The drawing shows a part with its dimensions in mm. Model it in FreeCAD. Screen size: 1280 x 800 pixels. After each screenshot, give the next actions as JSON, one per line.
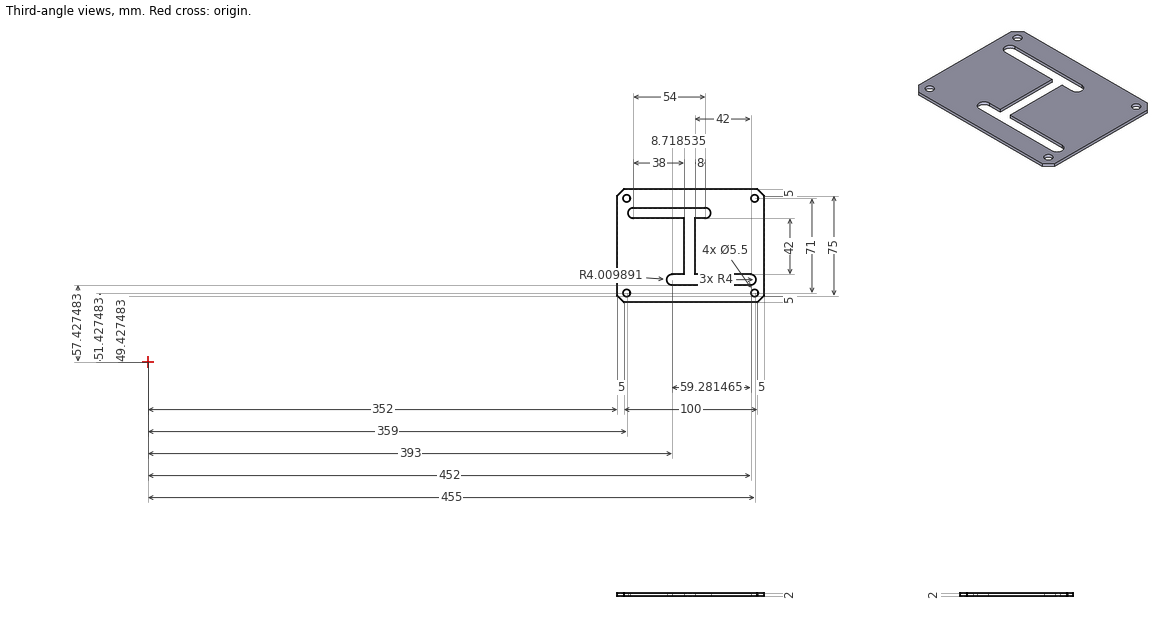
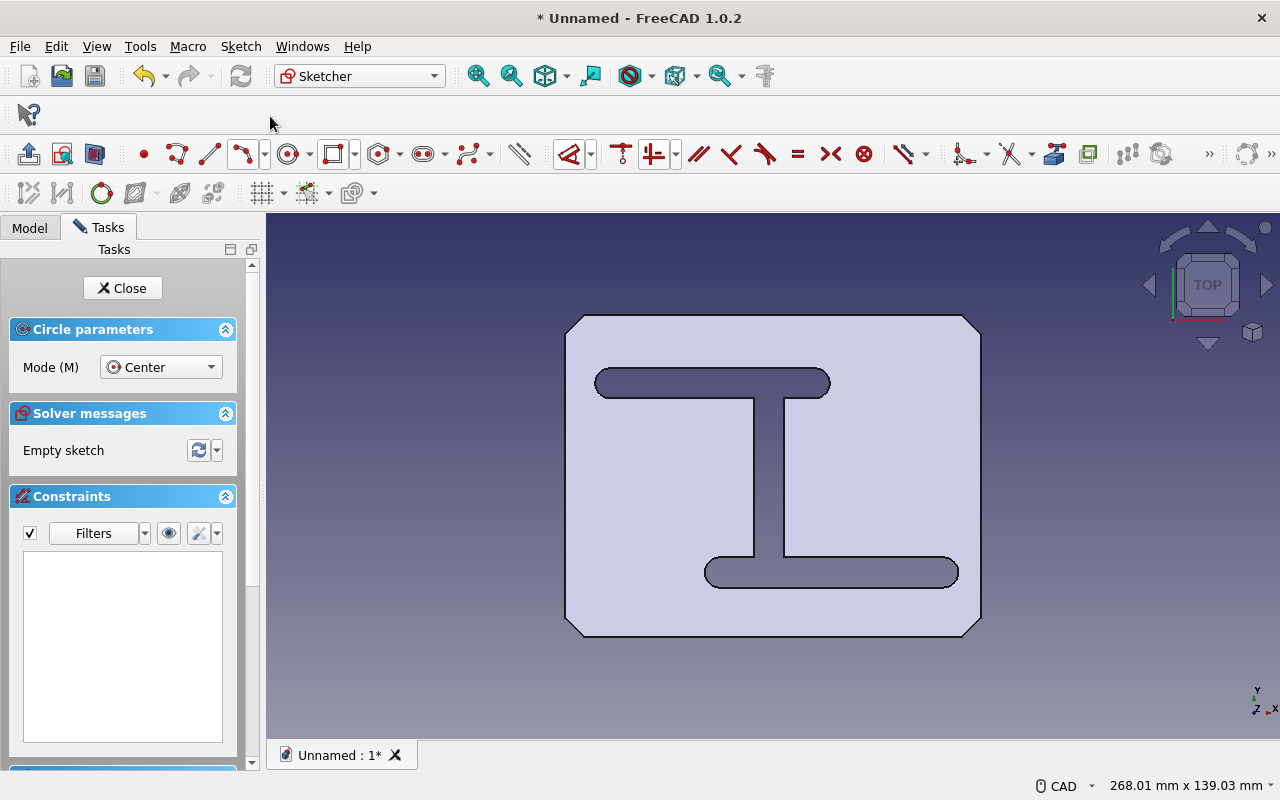
{"action": "scroll", "coordinate": [955, 610], "scroll_direction": "up", "scroll_amount": 4}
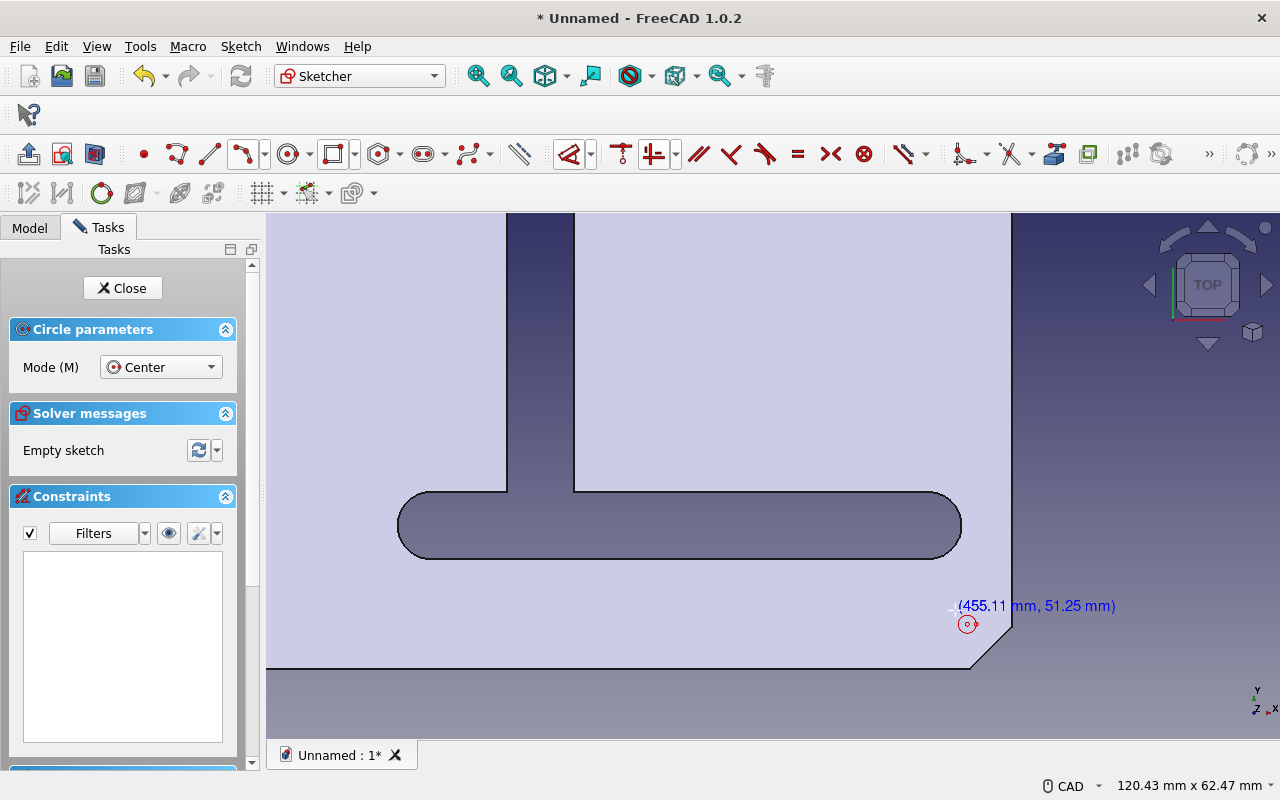
{"action": "left_click", "coordinate": [953, 610]}
{"action": "left_click", "coordinate": [970, 593]}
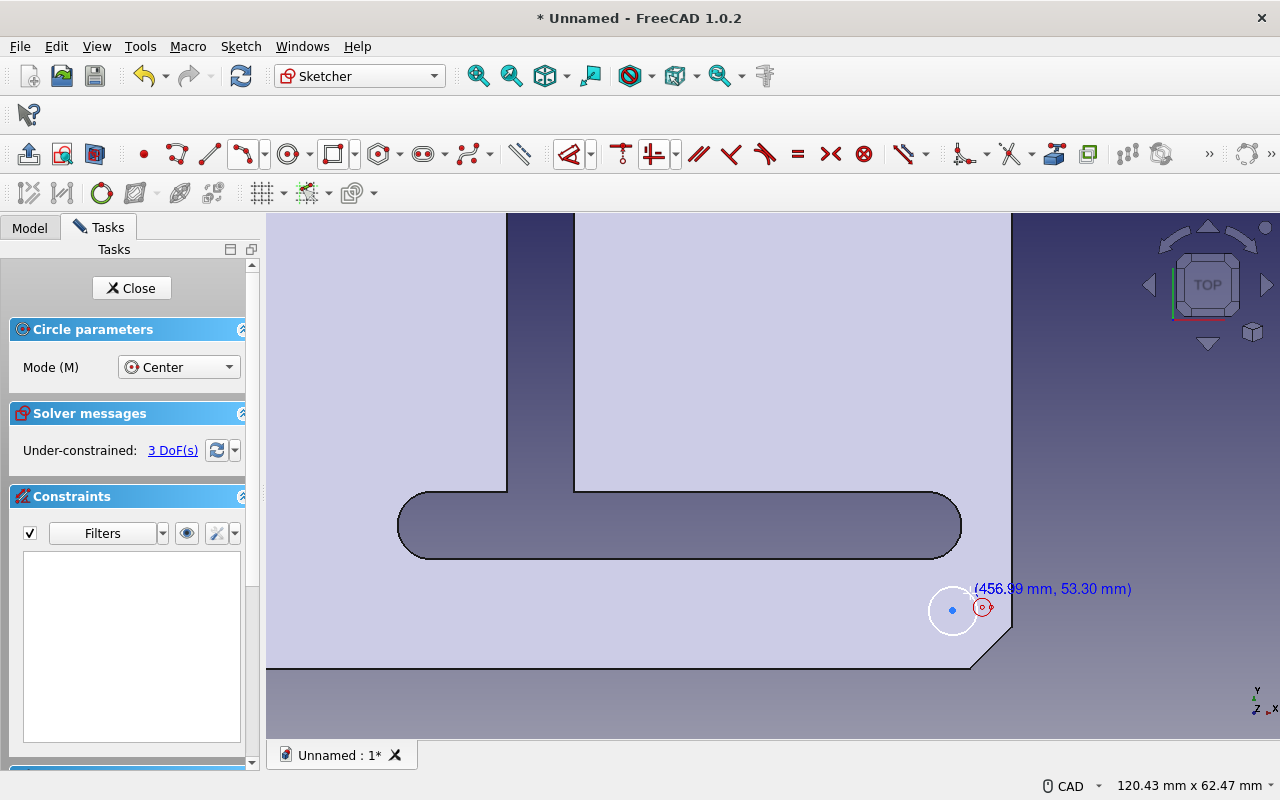
{"action": "scroll", "coordinate": [894, 677], "scroll_direction": "down", "scroll_amount": 3}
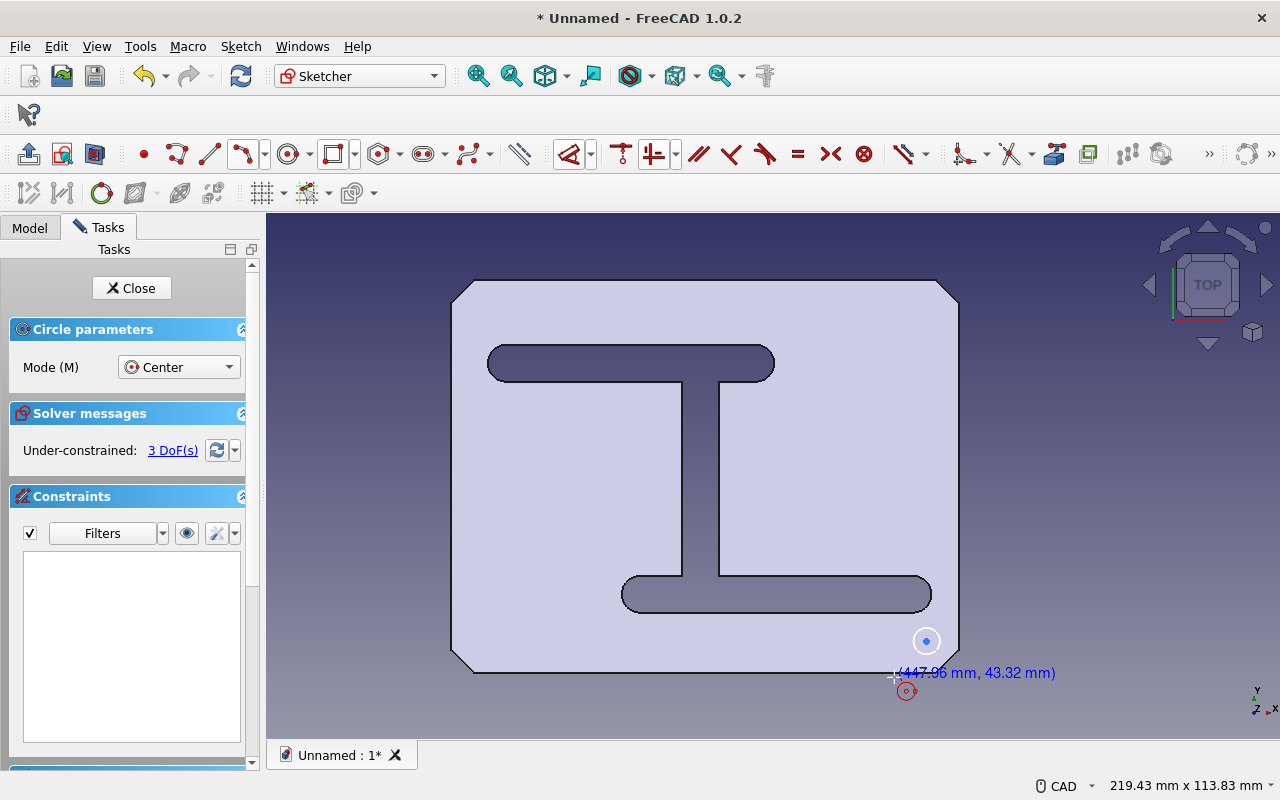
{"action": "scroll", "coordinate": [483, 640], "scroll_direction": "up", "scroll_amount": 3}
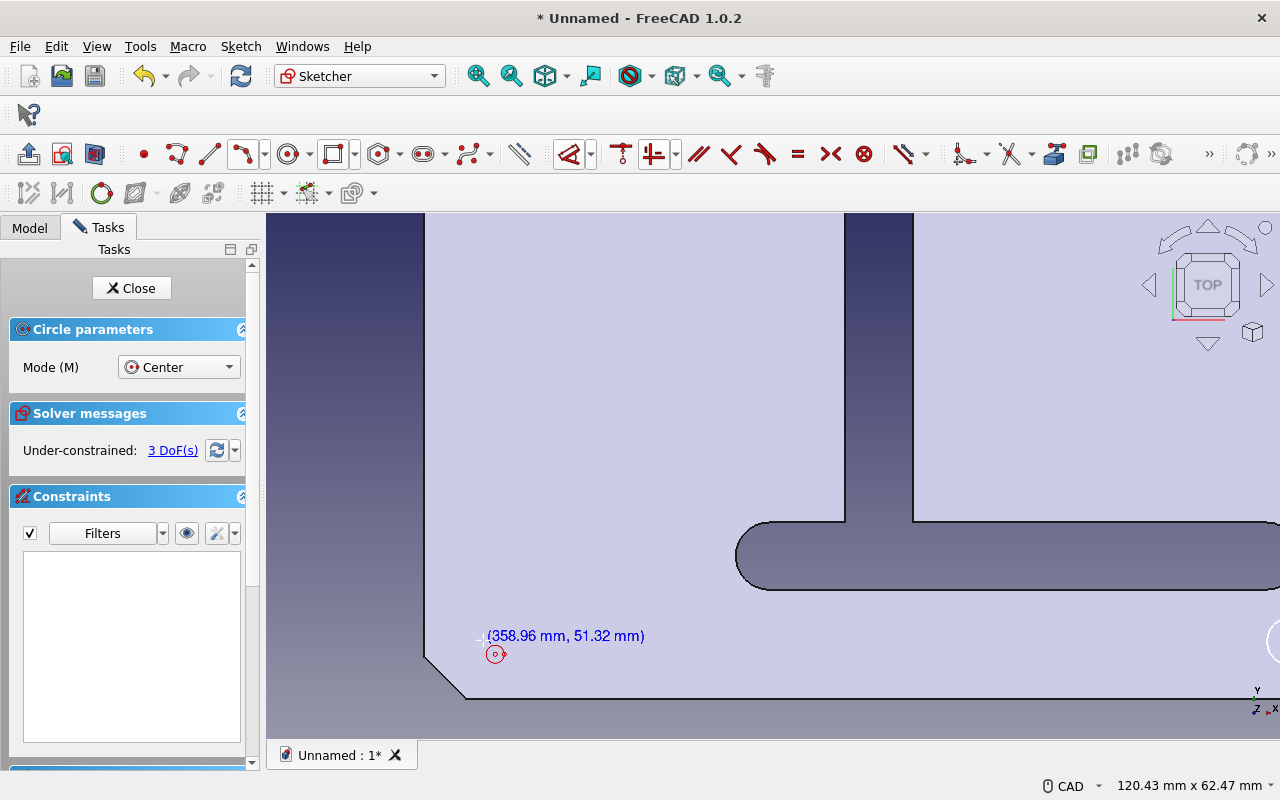
{"action": "left_click", "coordinate": [483, 640]}
{"action": "left_click", "coordinate": [500, 624]}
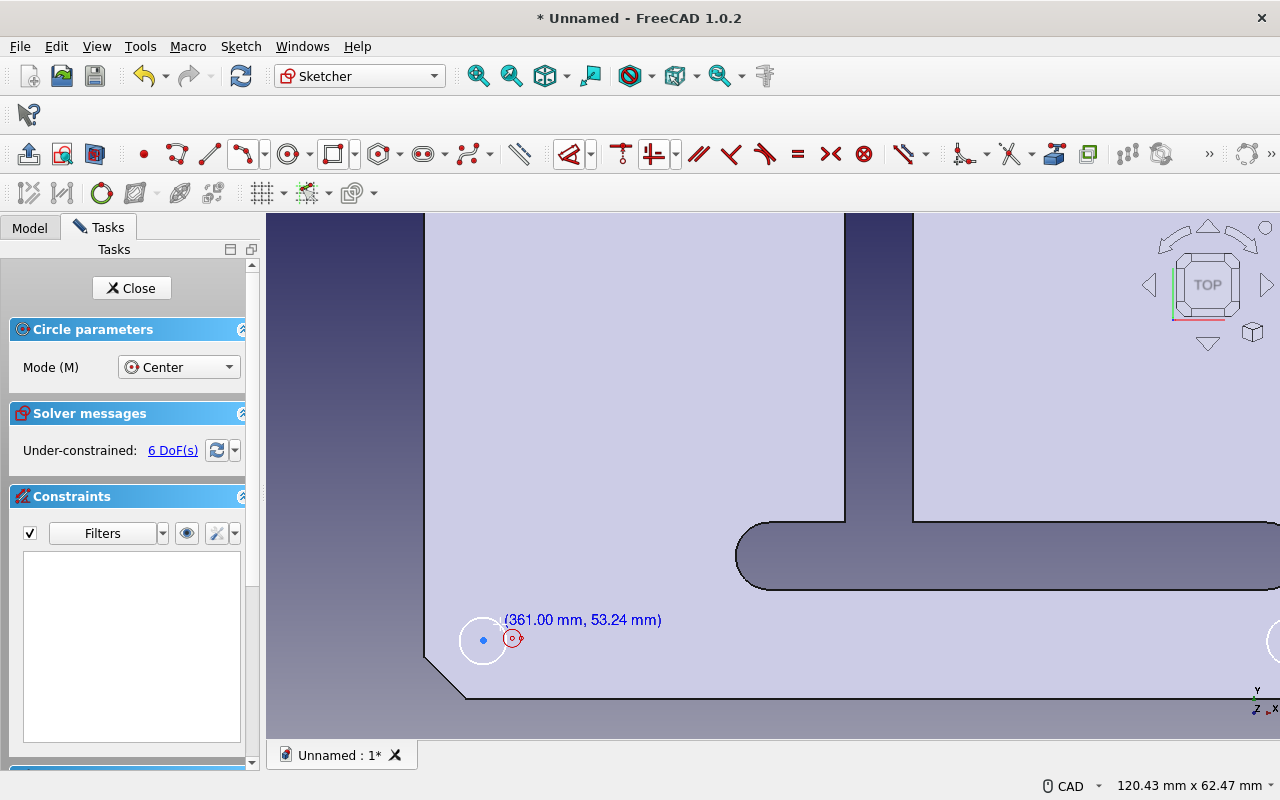
{"action": "scroll", "coordinate": [482, 640], "scroll_direction": "down", "scroll_amount": 3}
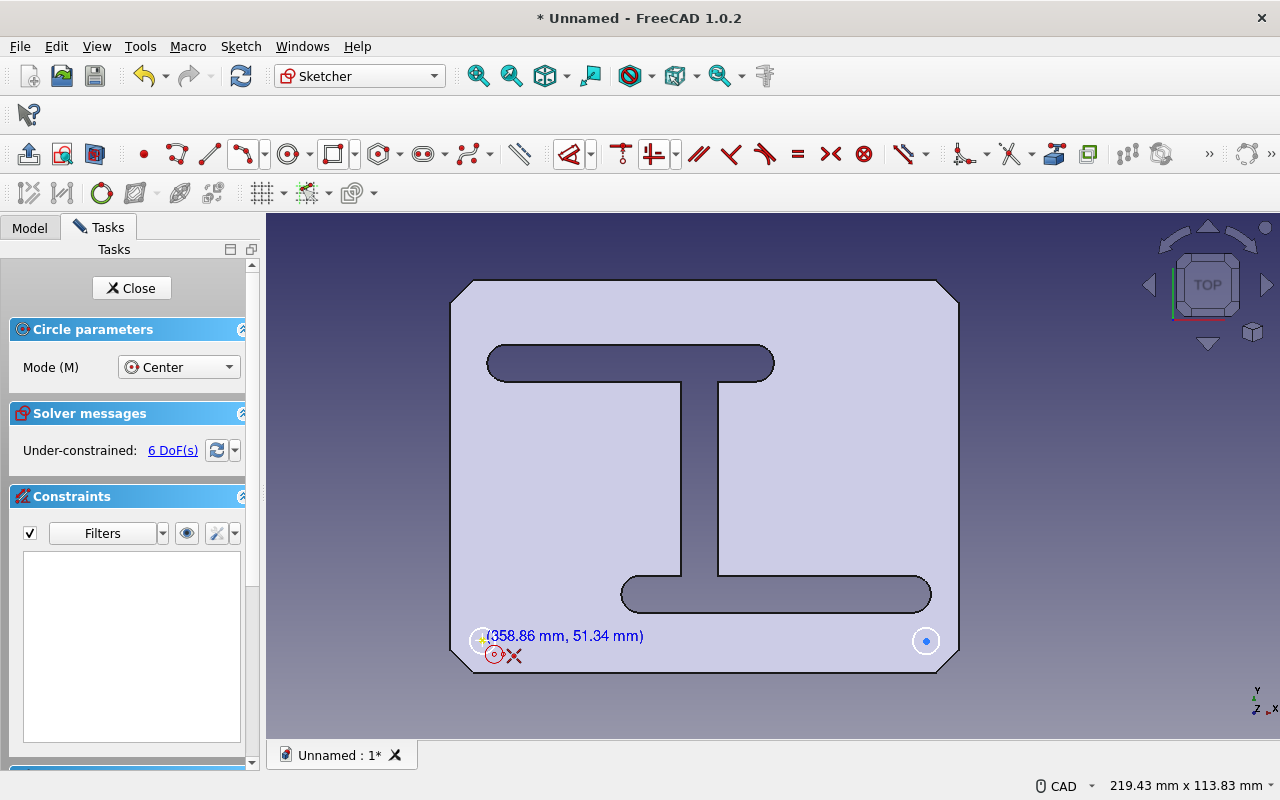
{"action": "scroll", "coordinate": [926, 312], "scroll_direction": "up", "scroll_amount": 3}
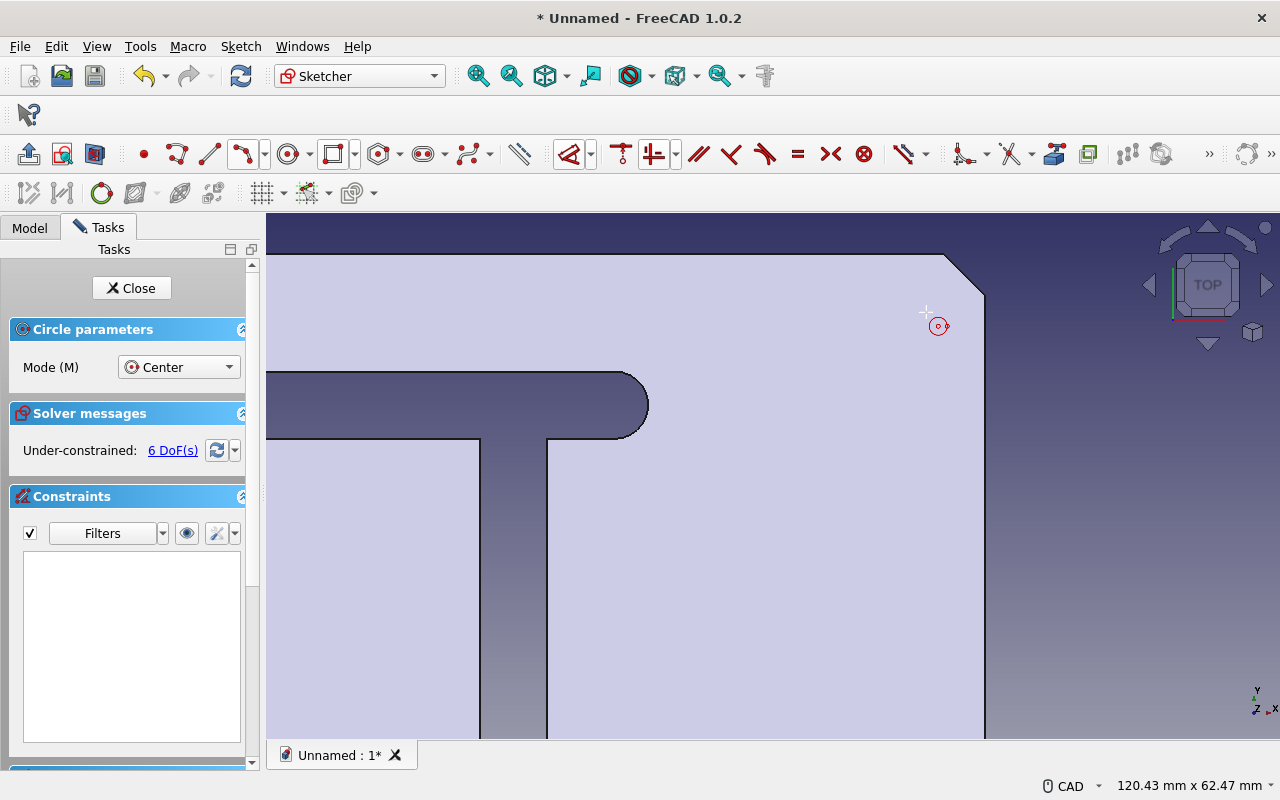
{"action": "left_click", "coordinate": [926, 313]}
{"action": "left_click", "coordinate": [942, 296]}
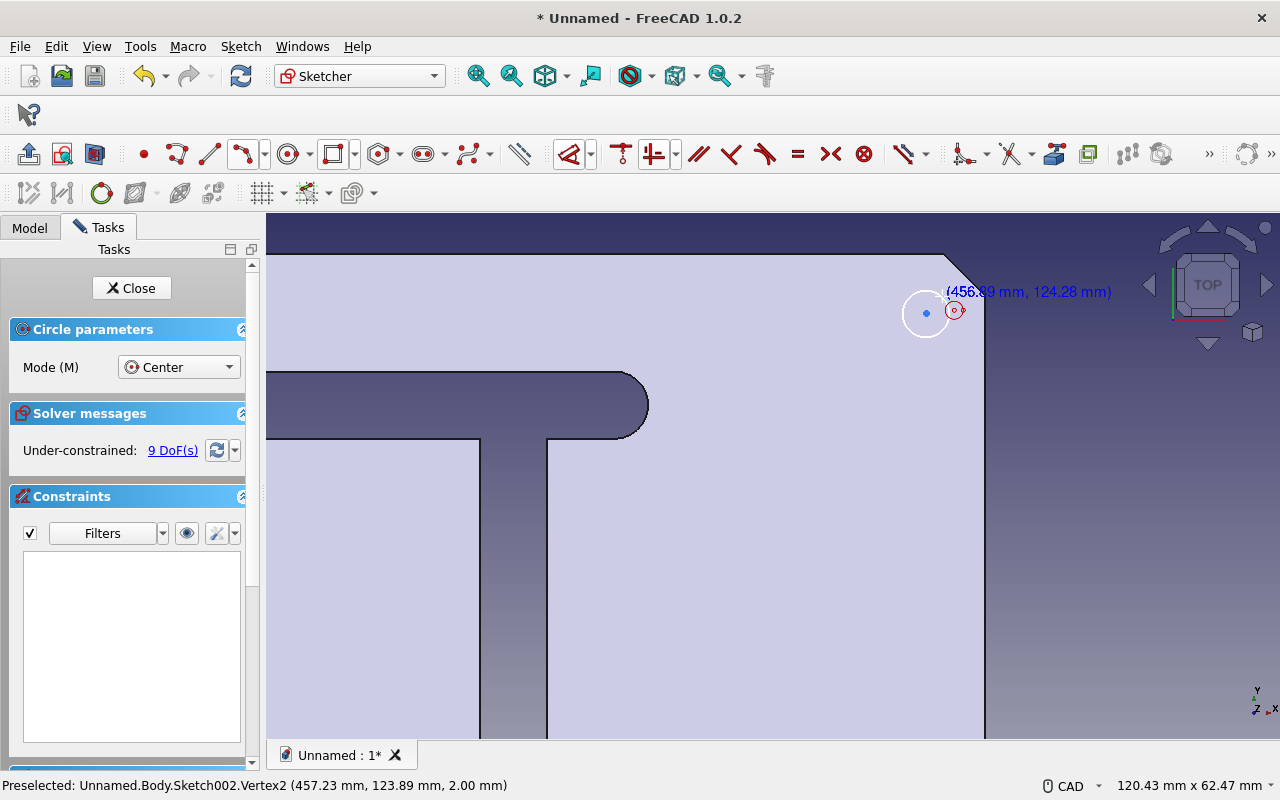
{"action": "scroll", "coordinate": [927, 311], "scroll_direction": "down", "scroll_amount": 3}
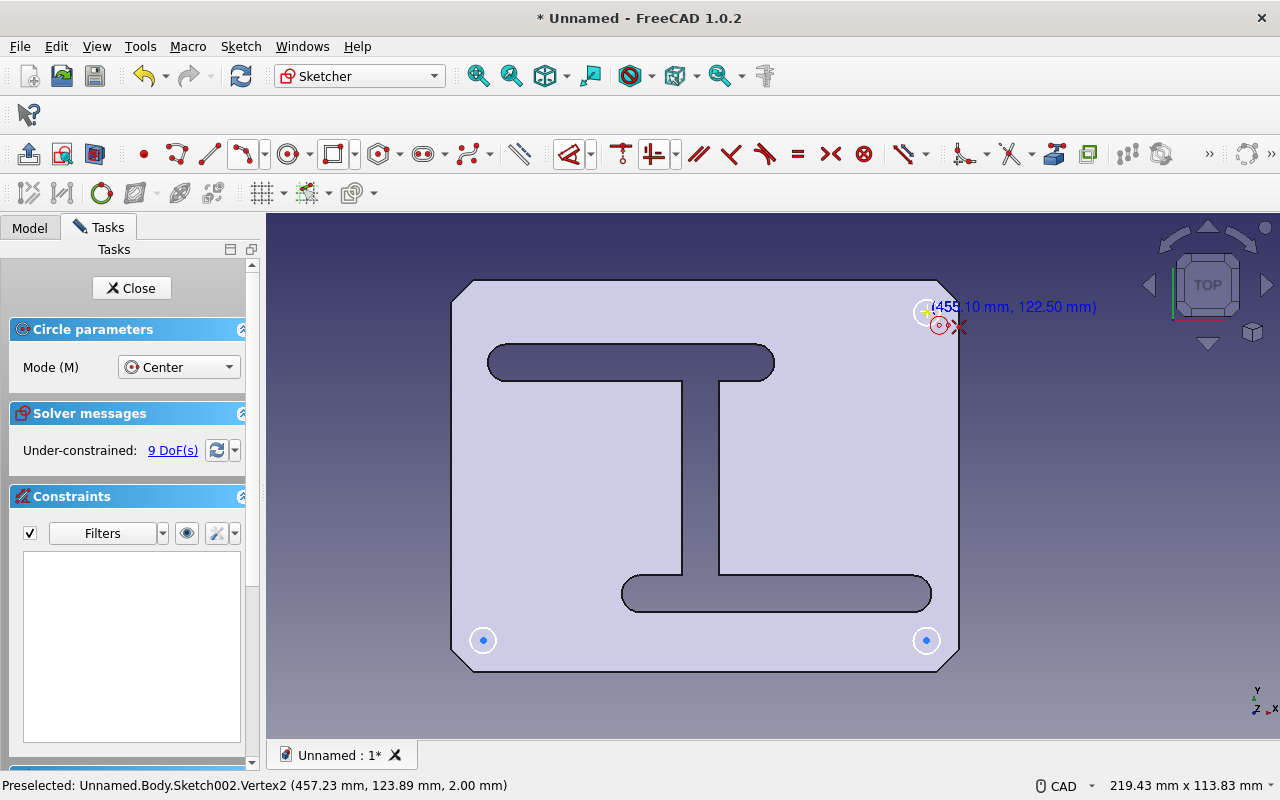
{"action": "scroll", "coordinate": [483, 312], "scroll_direction": "up", "scroll_amount": 3}